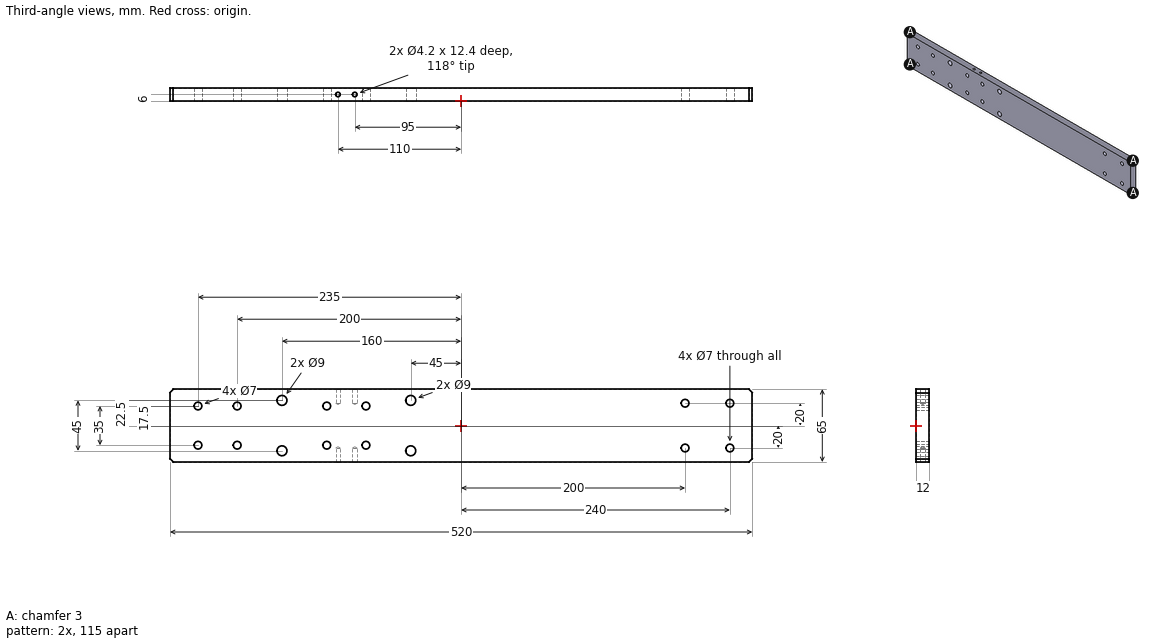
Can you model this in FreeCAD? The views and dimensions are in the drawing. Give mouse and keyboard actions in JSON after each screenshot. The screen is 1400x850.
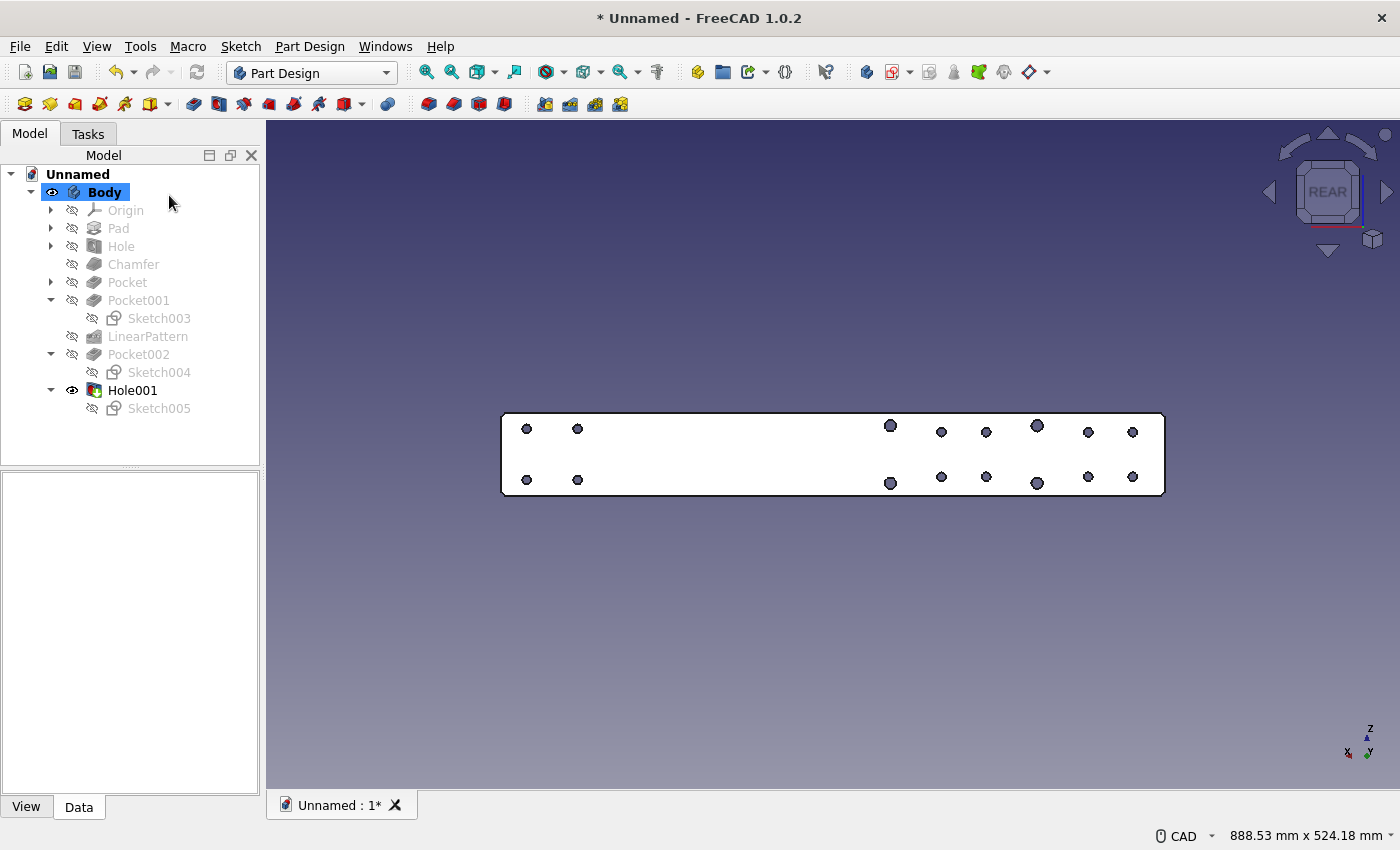
{"action": "left_click", "coordinate": [51, 210]}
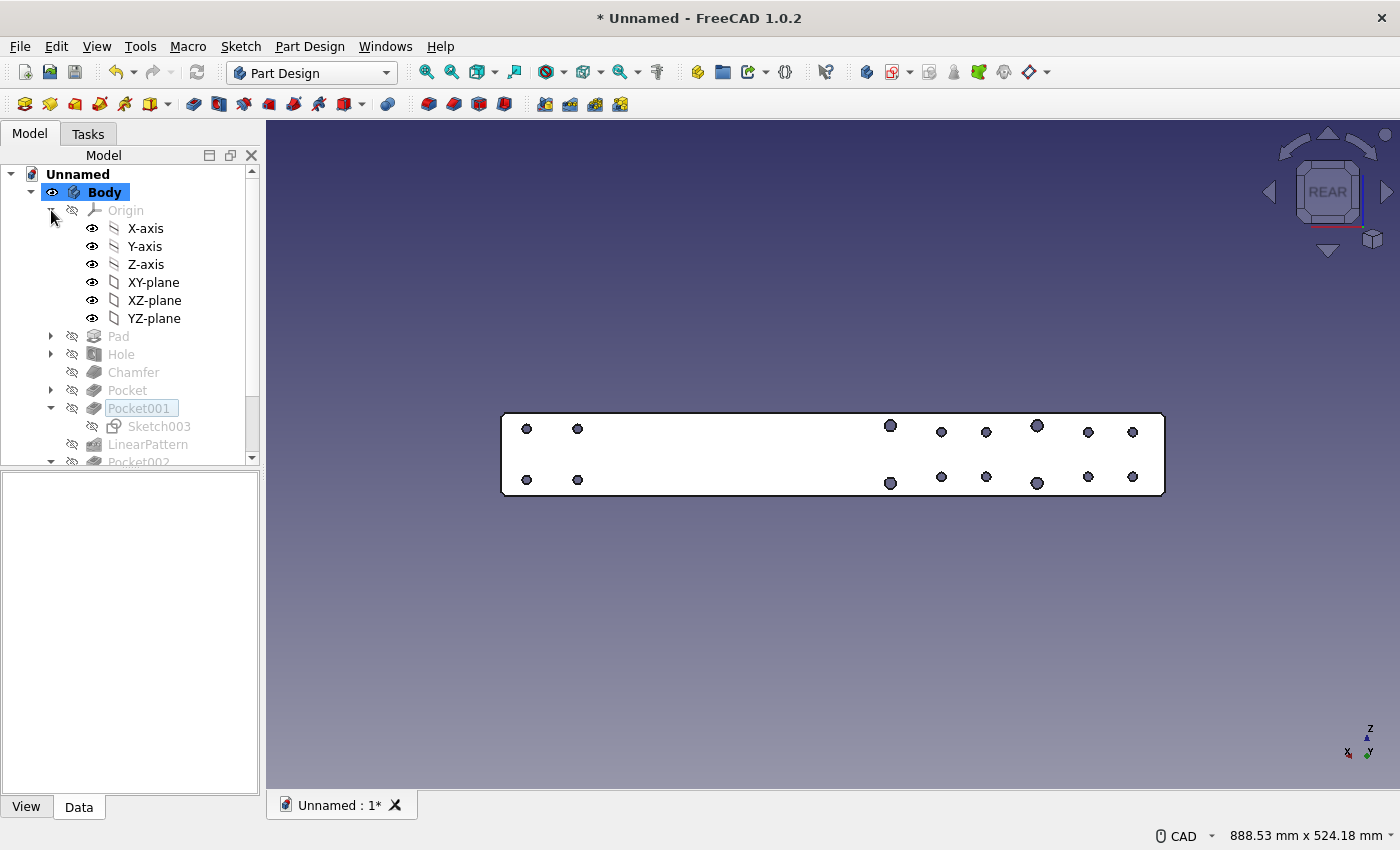
{"action": "left_click", "coordinate": [137, 282]}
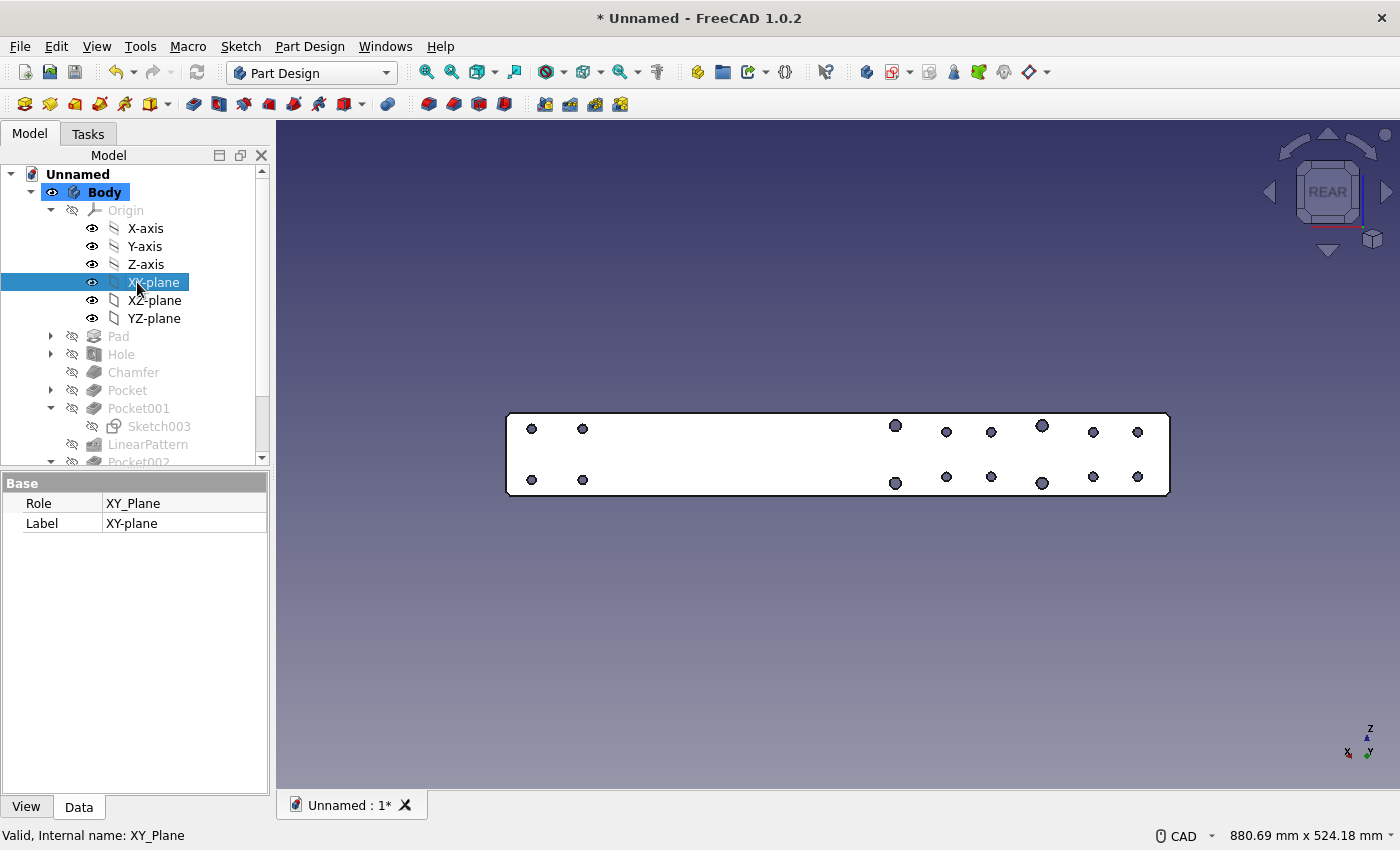
{"action": "left_click", "coordinate": [1028, 72]}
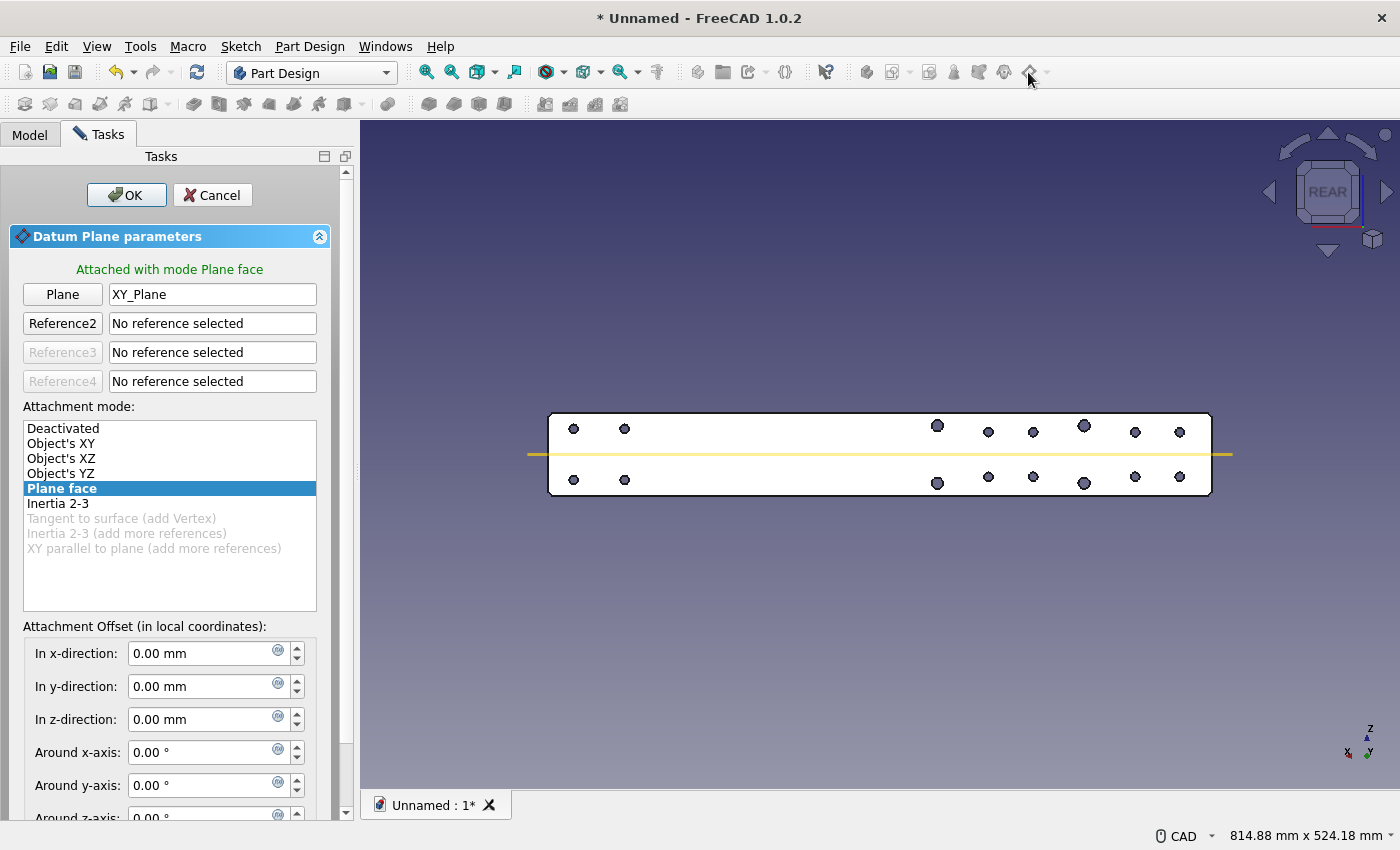
{"action": "triple_click", "coordinate": [210, 720]}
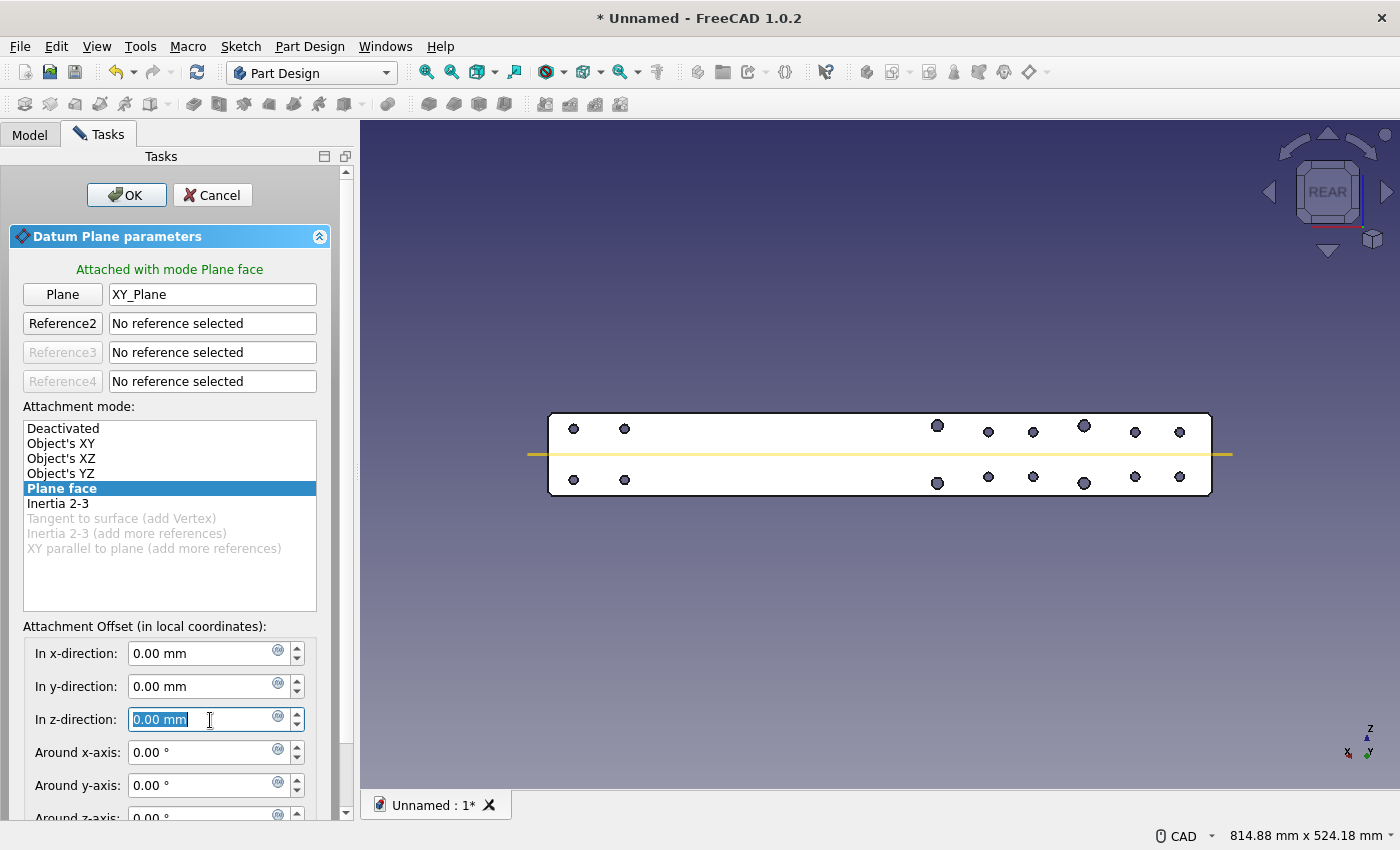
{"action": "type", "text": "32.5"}
{"action": "key", "text": "Tab"}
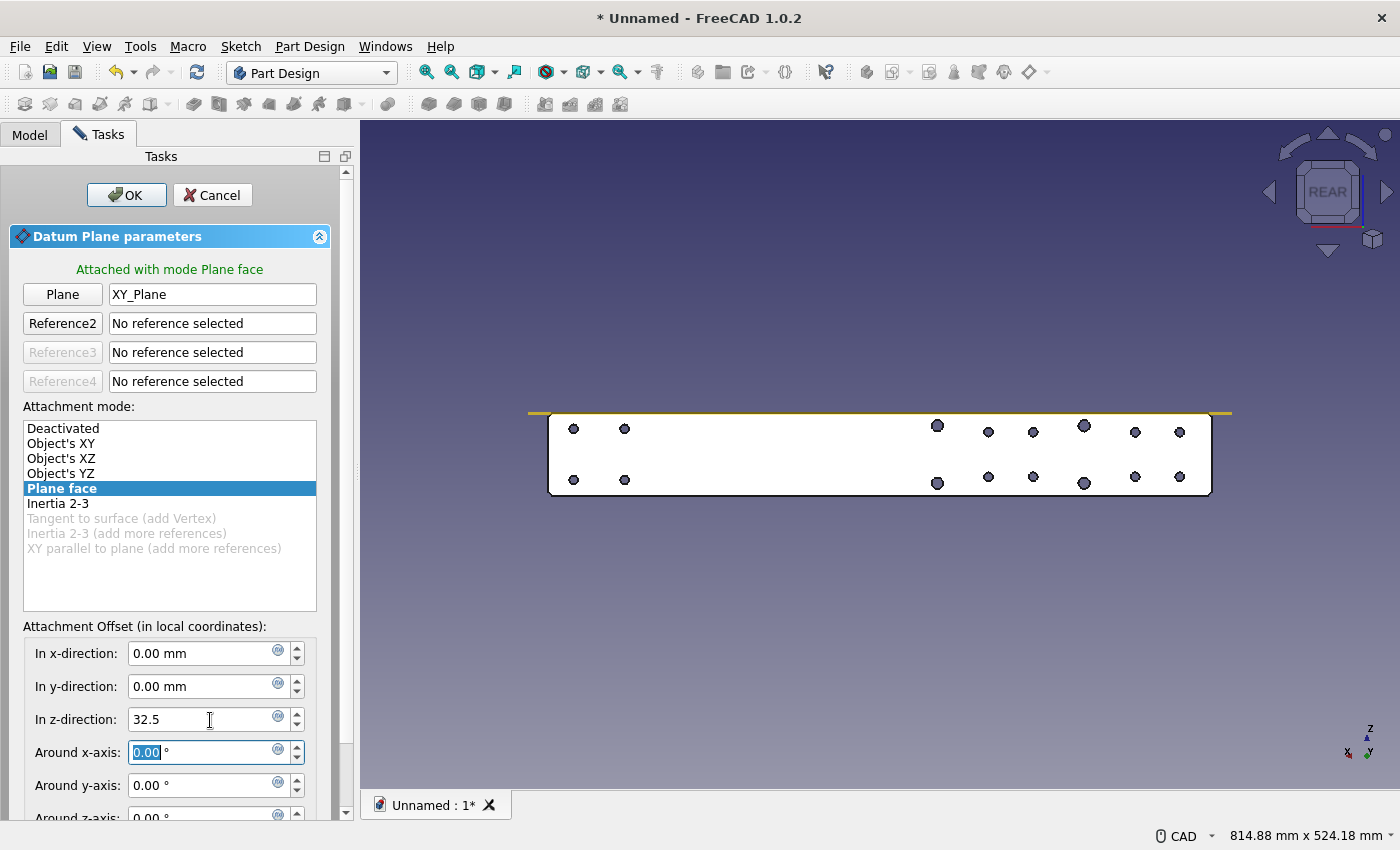
{"action": "left_click", "coordinate": [127, 195]}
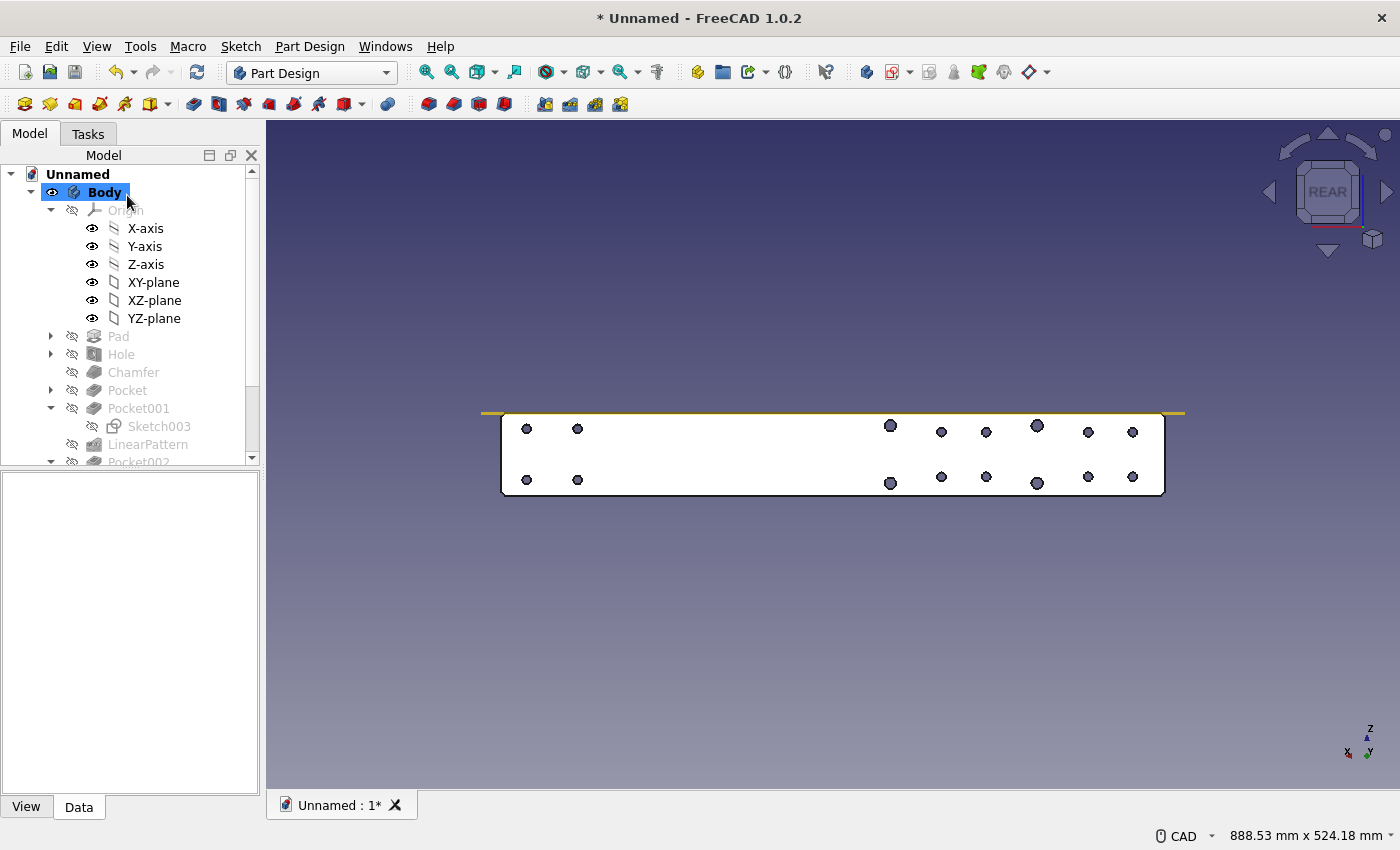
{"action": "scroll", "coordinate": [101, 314], "scroll_direction": "down", "scroll_amount": 3}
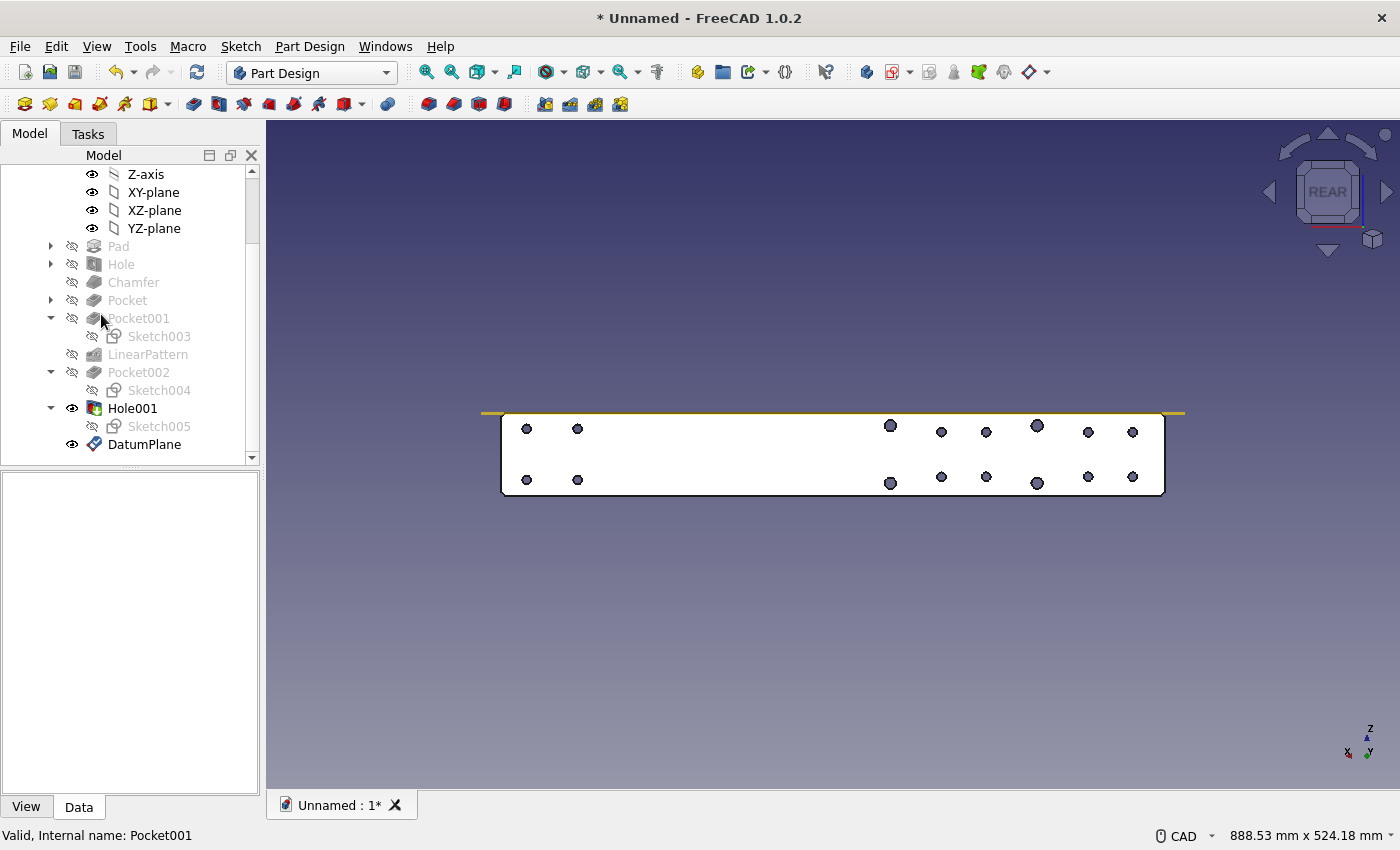
{"action": "left_click", "coordinate": [117, 444]}